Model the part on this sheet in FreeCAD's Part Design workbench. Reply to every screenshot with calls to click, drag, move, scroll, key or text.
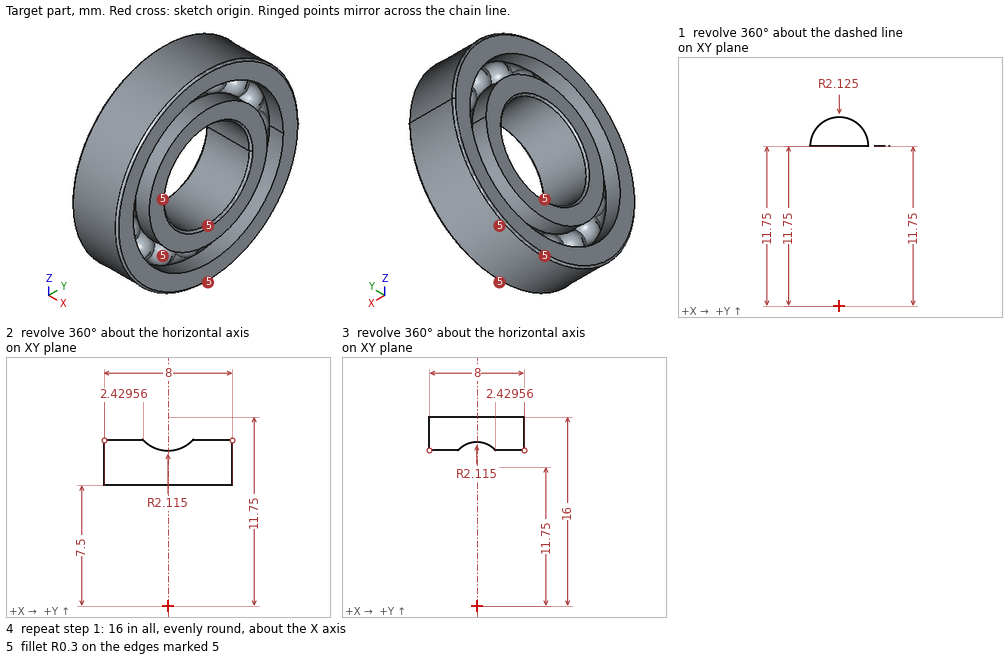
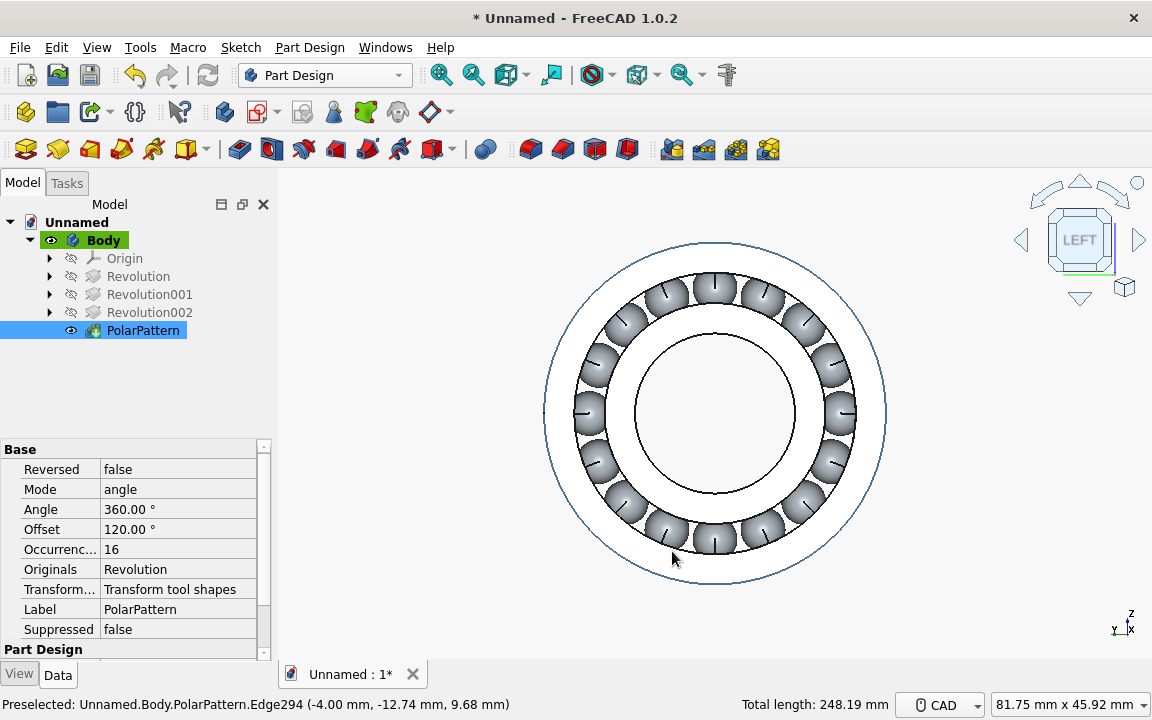
click(795, 412, ctrl)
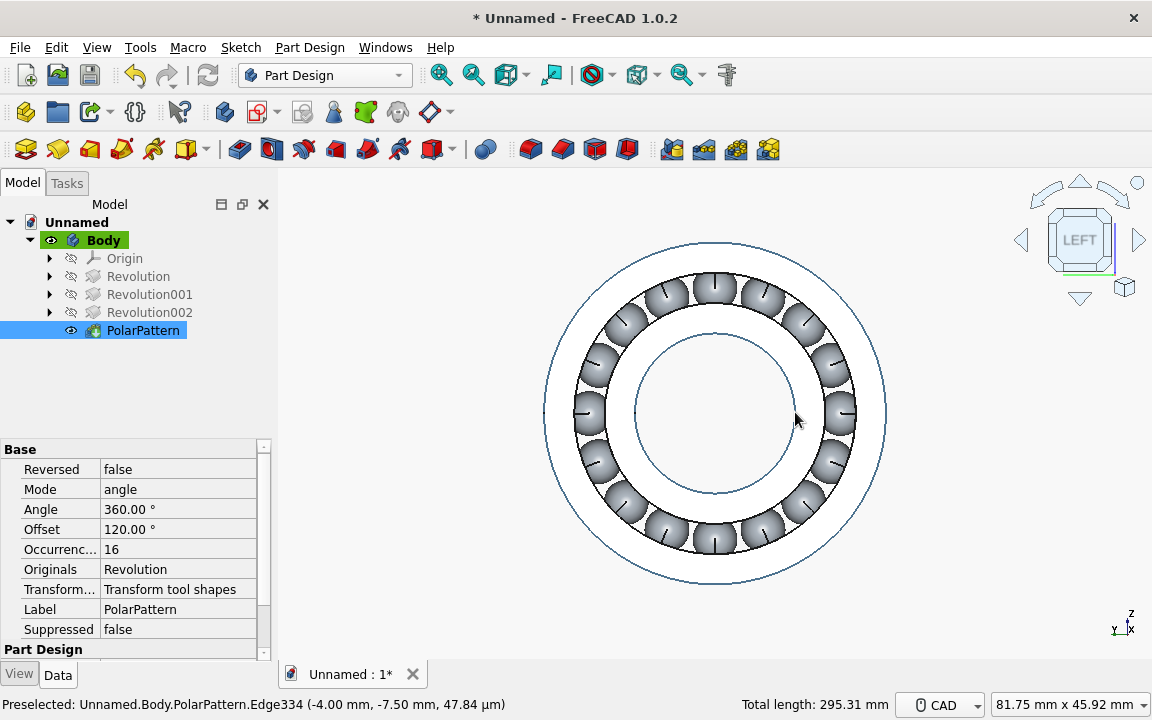
click(532, 150)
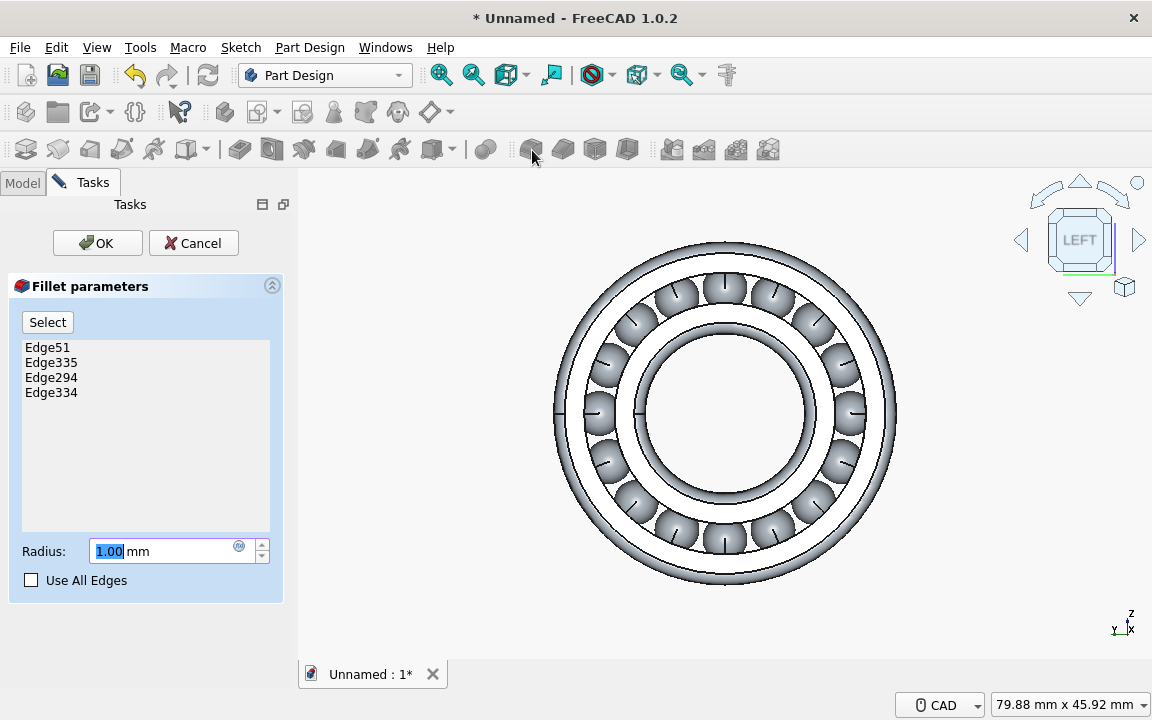
text(0.3)
key(Tab)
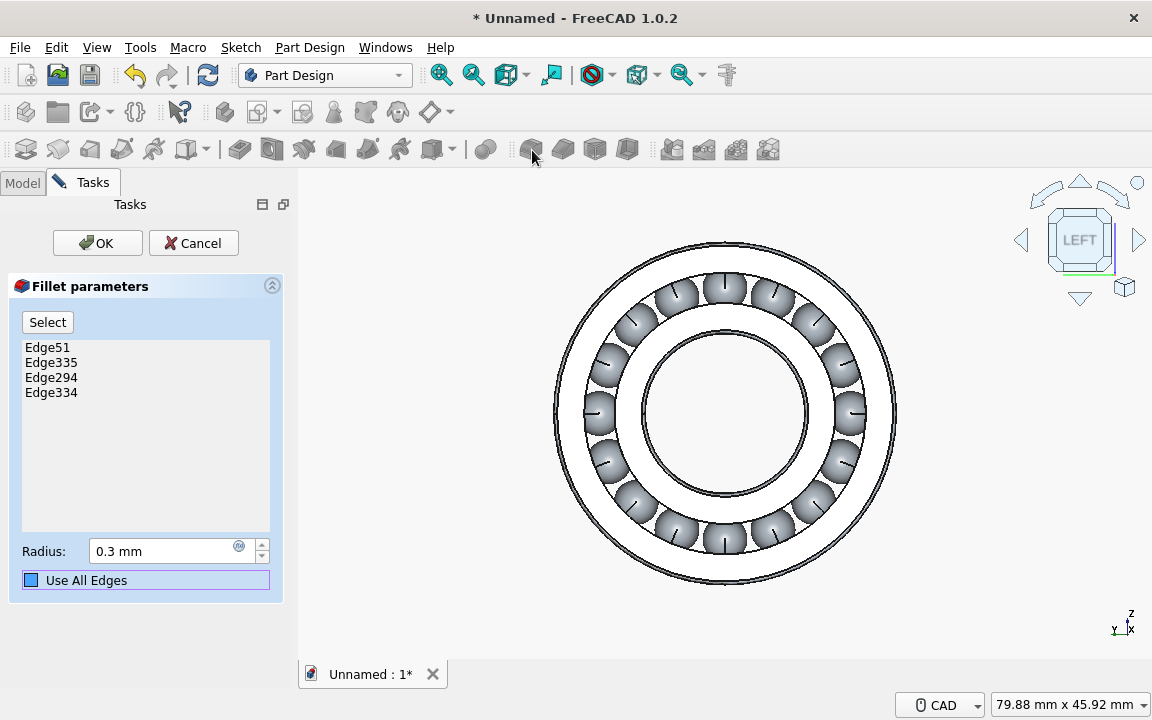
click(98, 243)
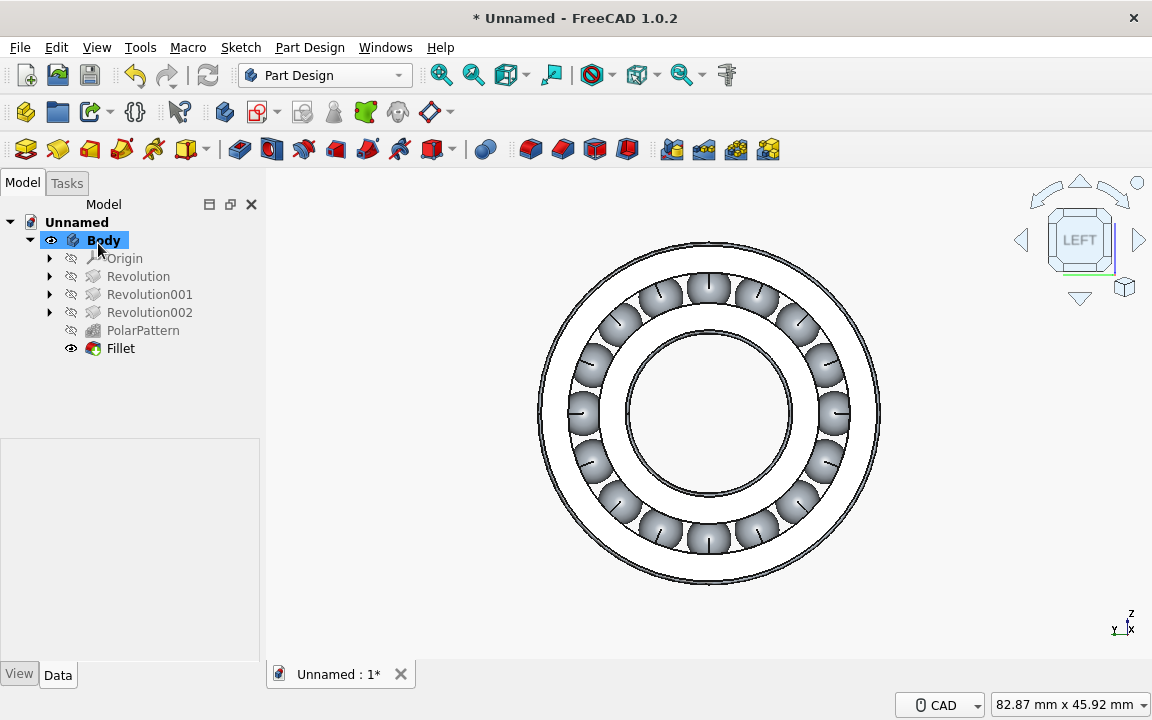
key(0)